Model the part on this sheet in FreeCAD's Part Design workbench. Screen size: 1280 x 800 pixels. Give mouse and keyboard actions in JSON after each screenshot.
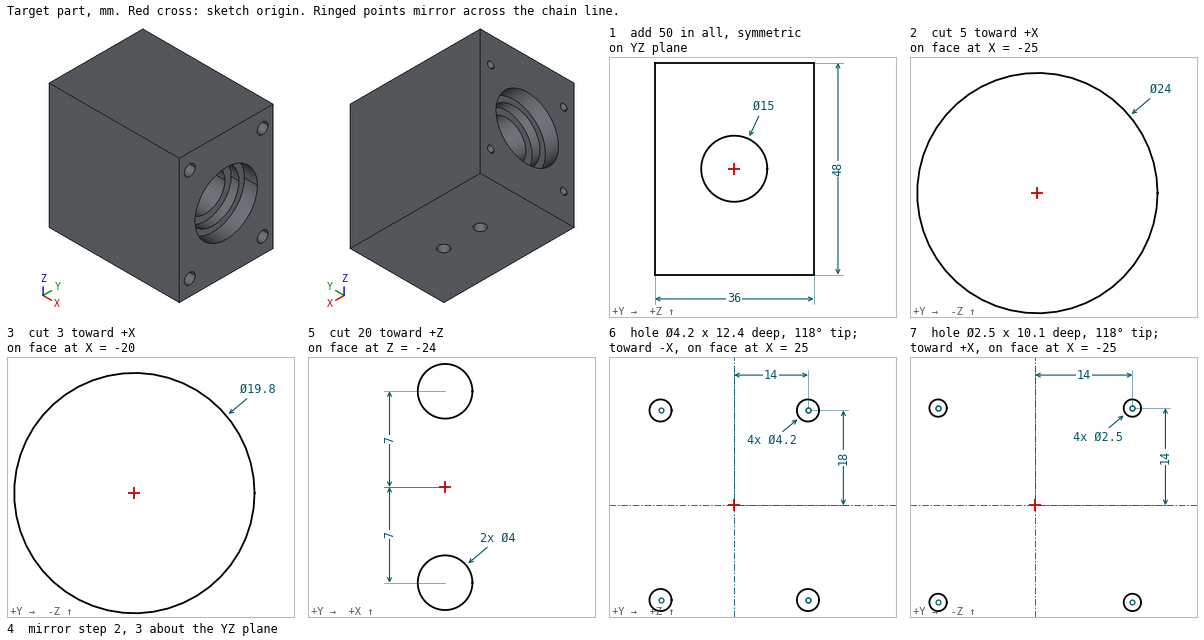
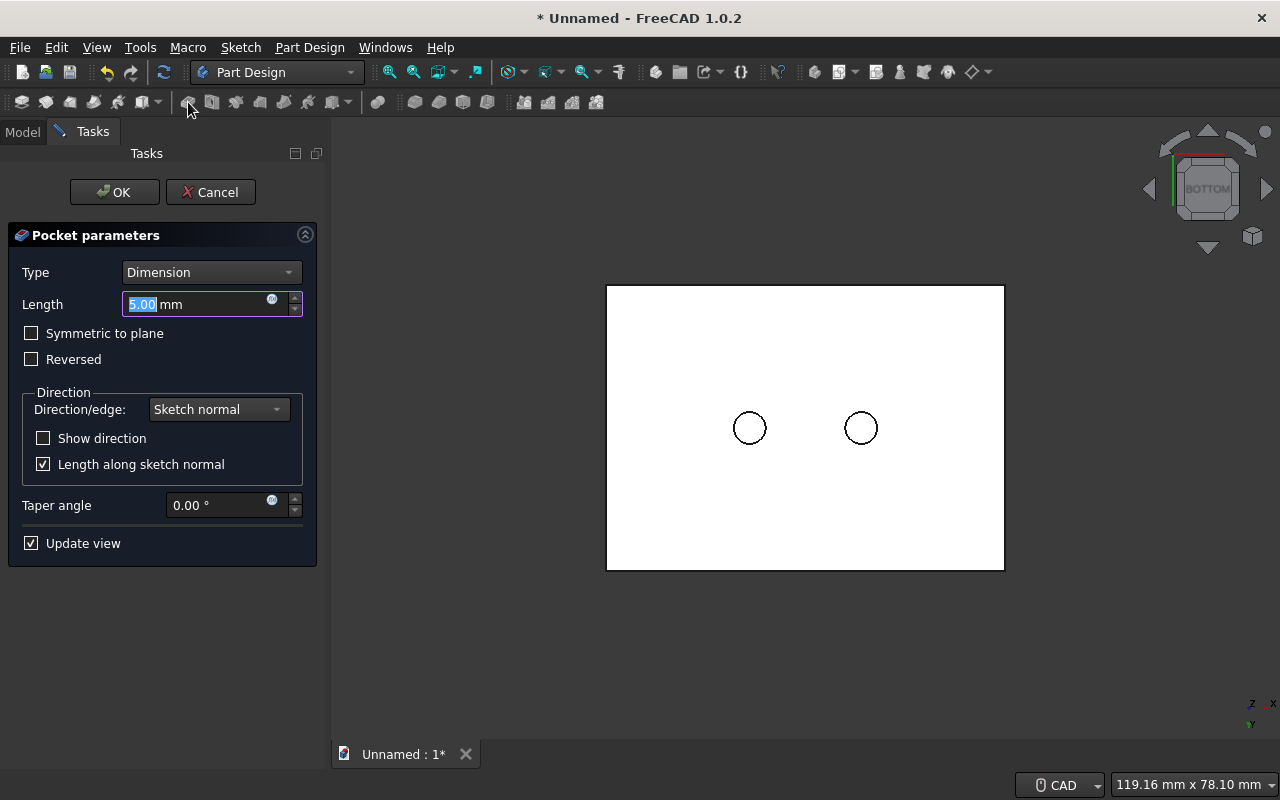
{"action": "type", "text": "20"}
{"action": "key", "text": "Tab"}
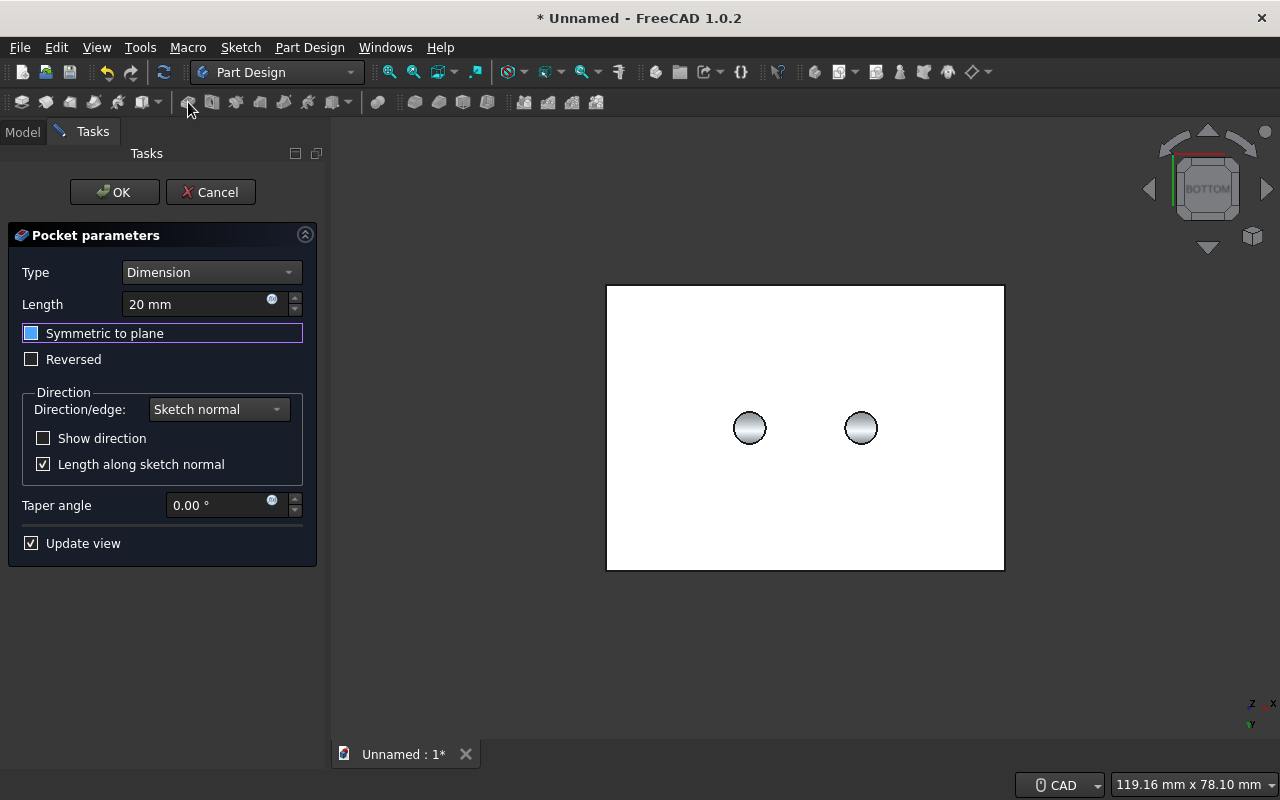
{"action": "left_click", "coordinate": [115, 192]}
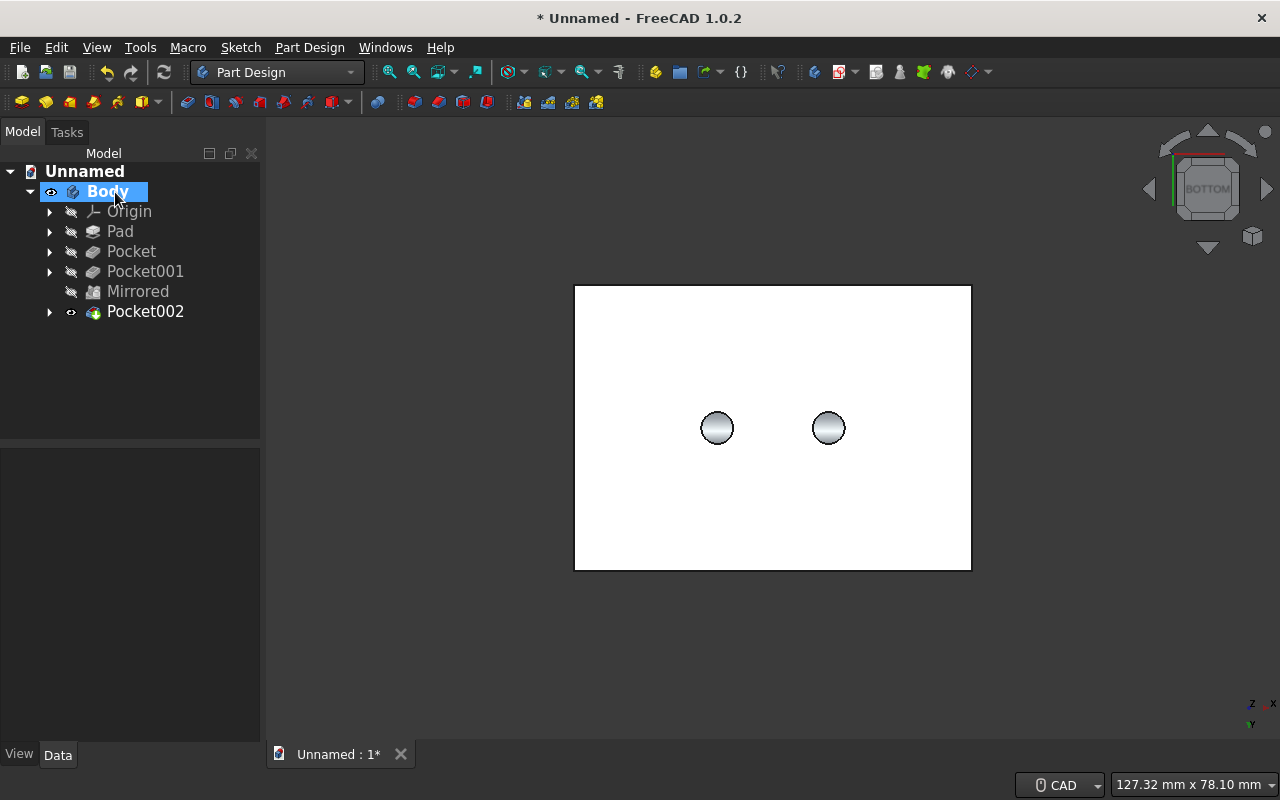
{"action": "key", "text": "0"}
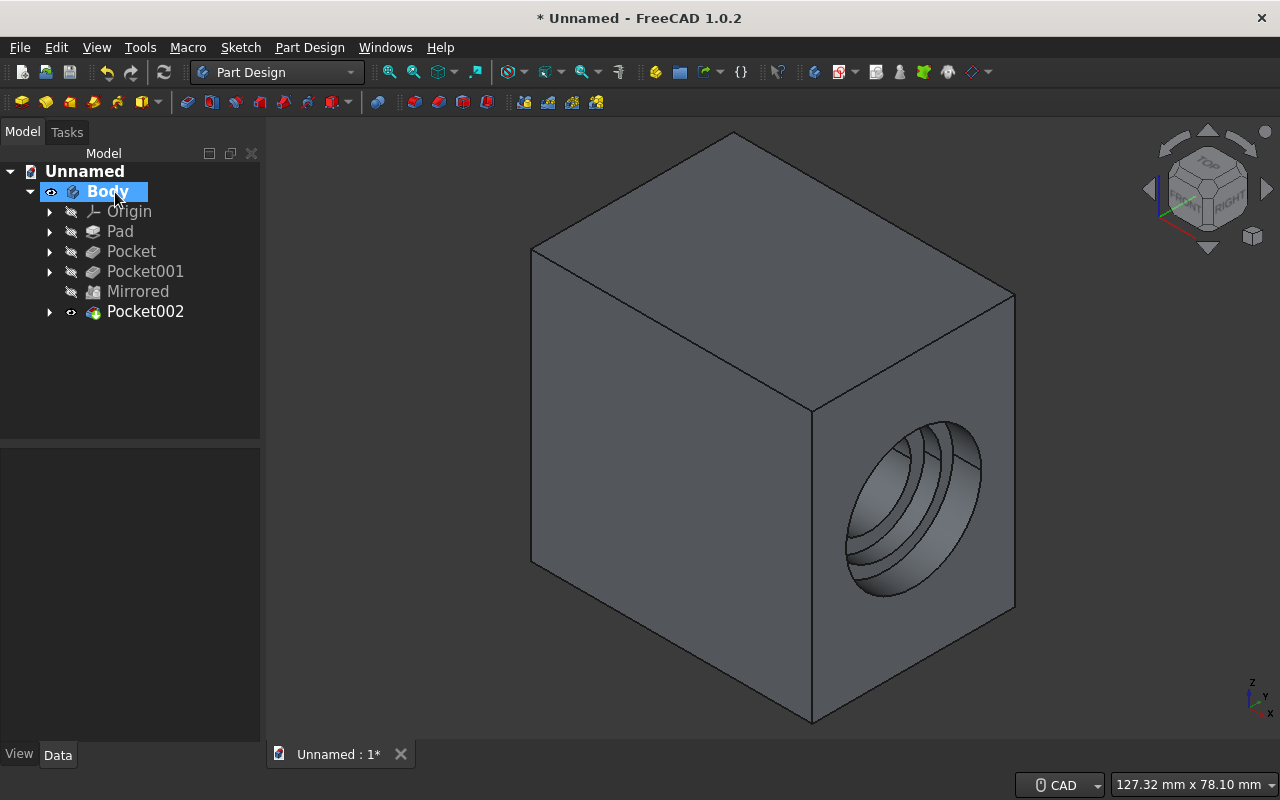
{"action": "left_click", "coordinate": [972, 386]}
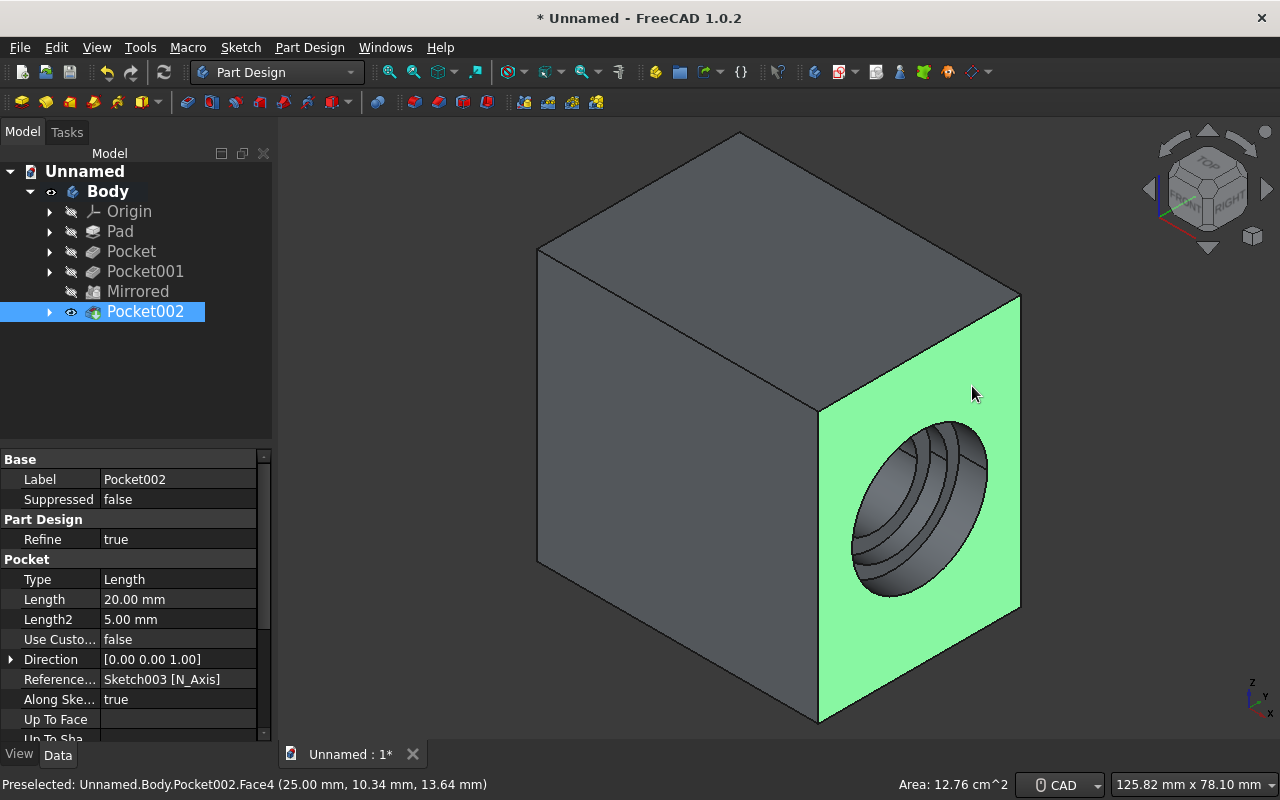
{"action": "left_click", "coordinate": [840, 72]}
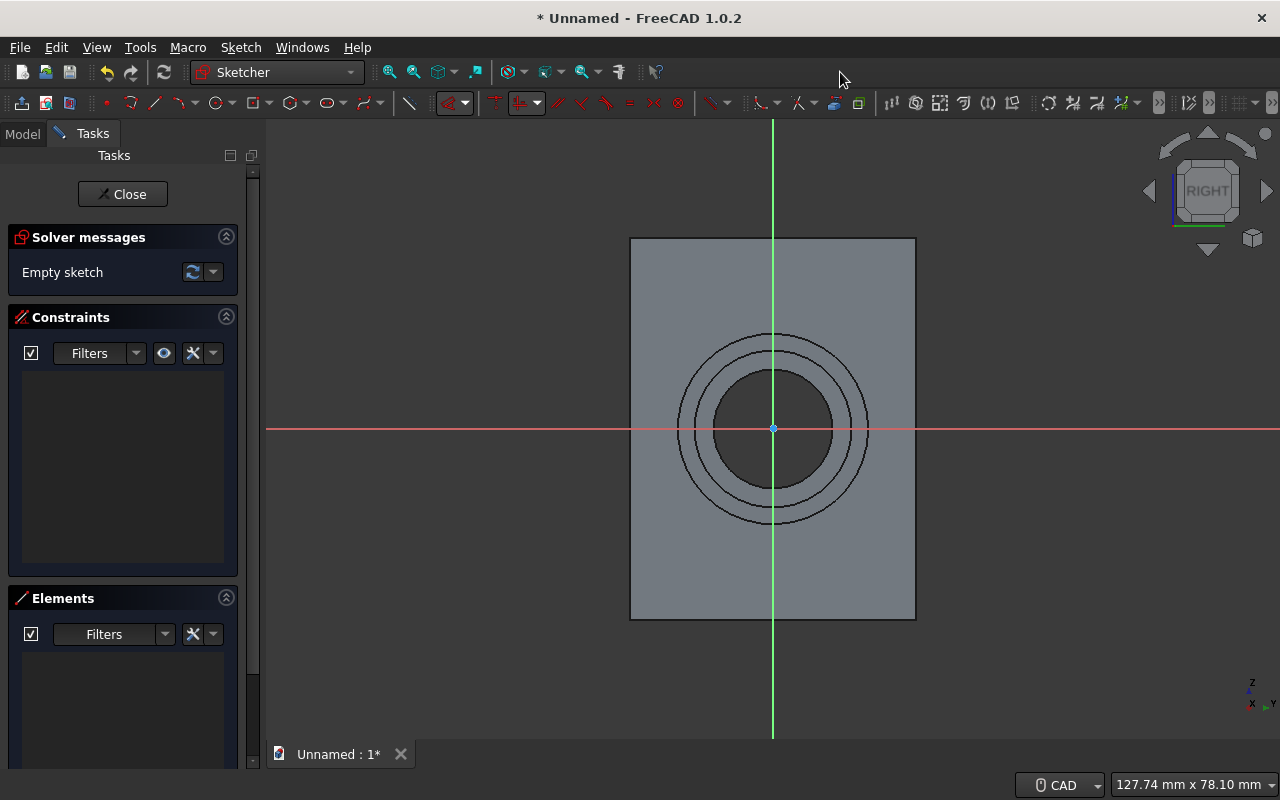
{"action": "left_click", "coordinate": [216, 104]}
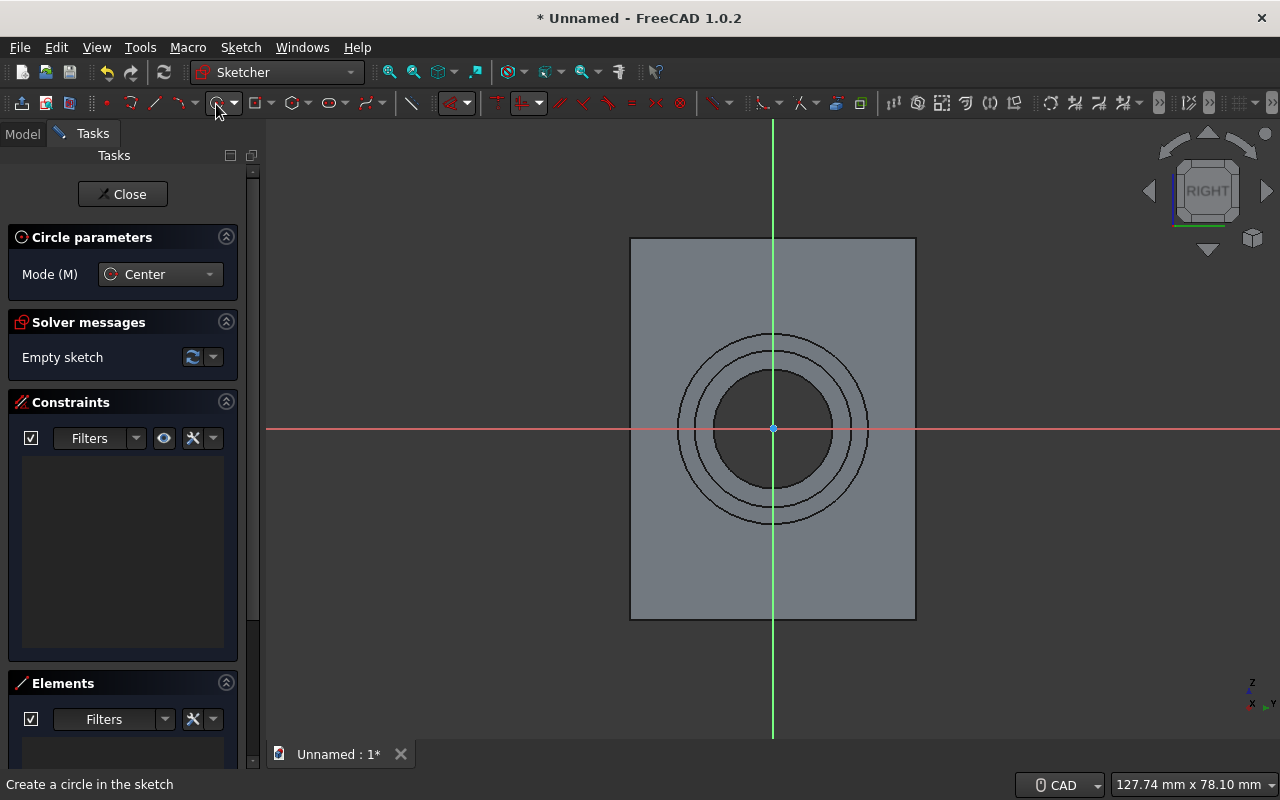
{"action": "scroll", "coordinate": [884, 286], "scroll_direction": "up", "scroll_amount": 2}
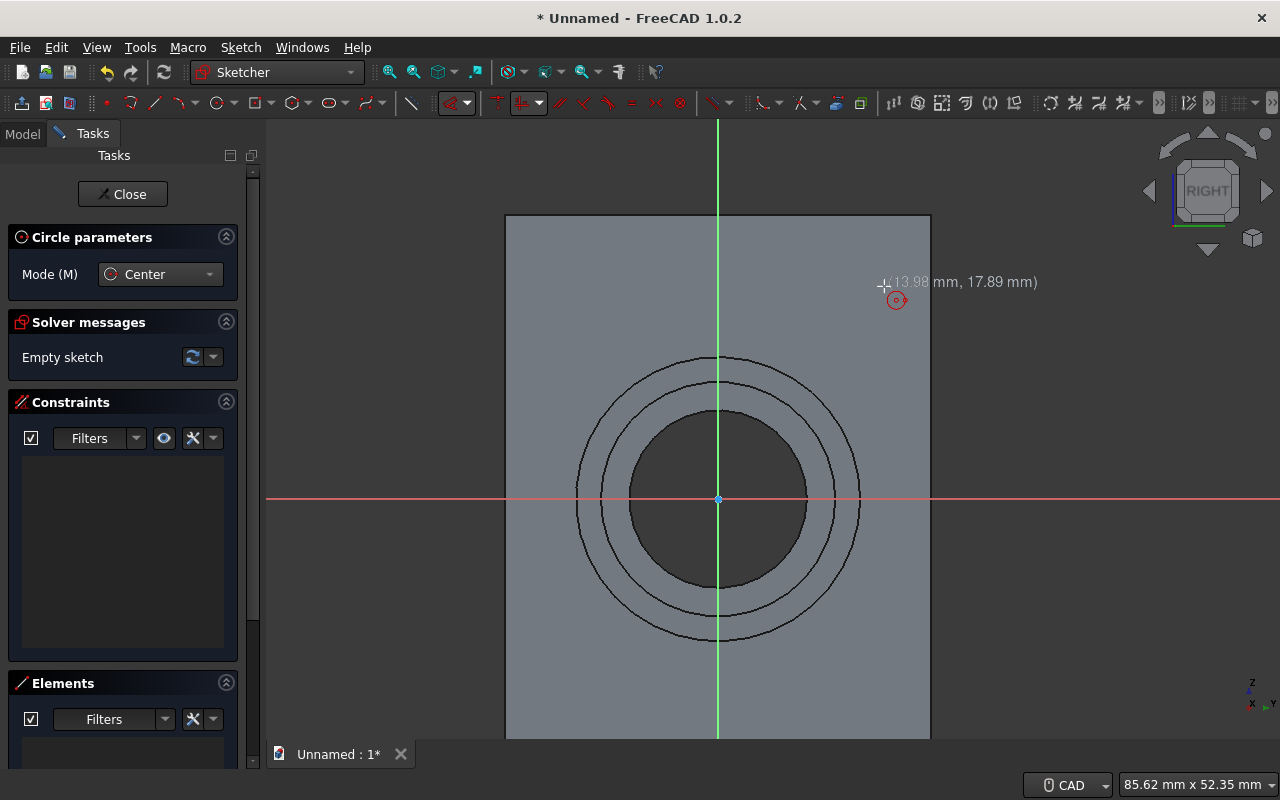
{"action": "left_click", "coordinate": [884, 286]}
{"action": "left_click", "coordinate": [901, 268]}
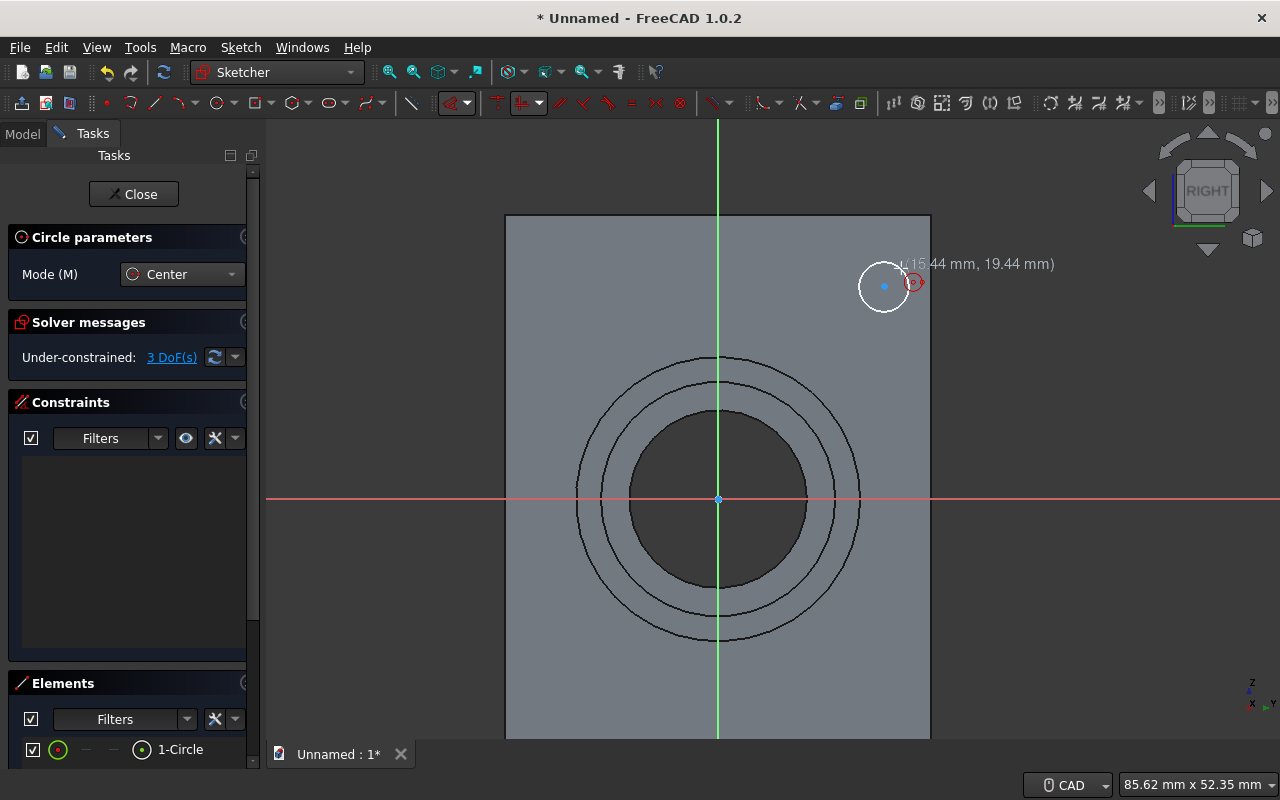
{"action": "scroll", "coordinate": [643, 147], "scroll_direction": "down", "scroll_amount": 1}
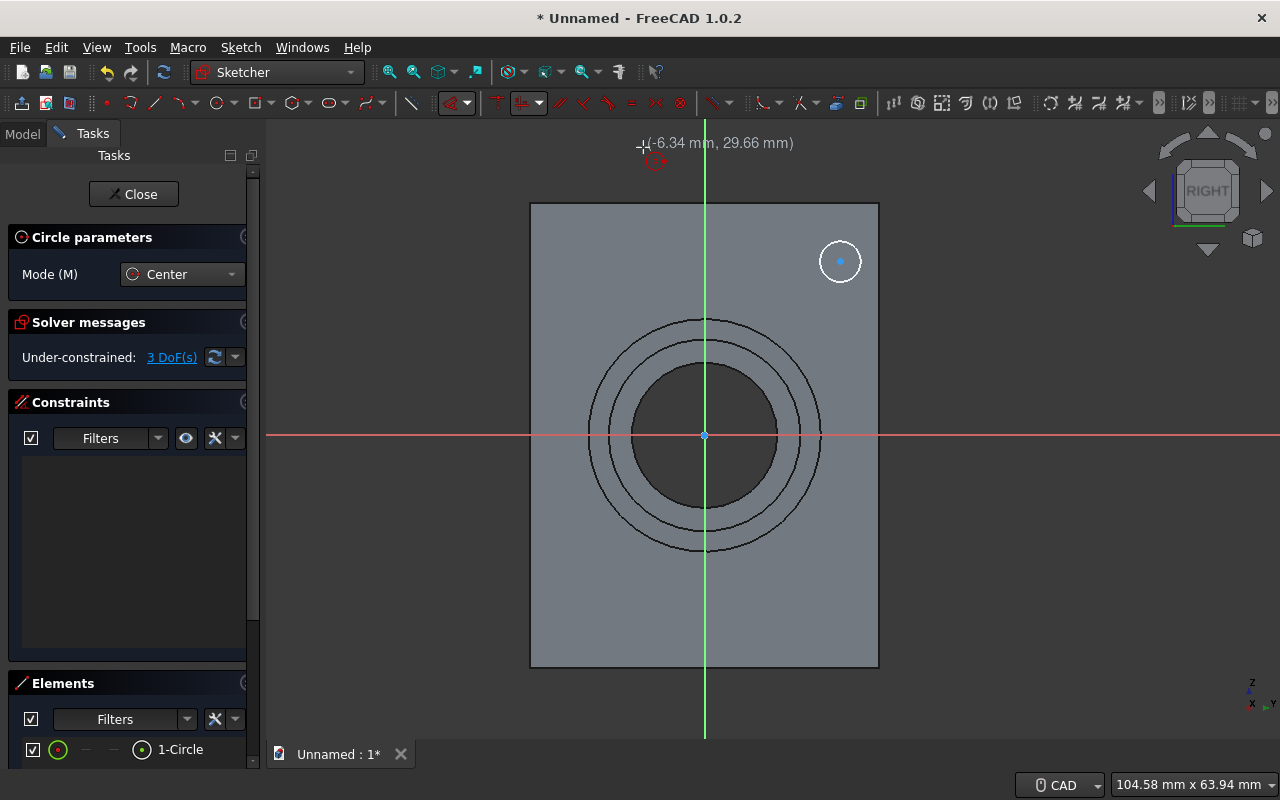
{"action": "left_click", "coordinate": [840, 610]}
{"action": "left_click", "coordinate": [855, 595]}